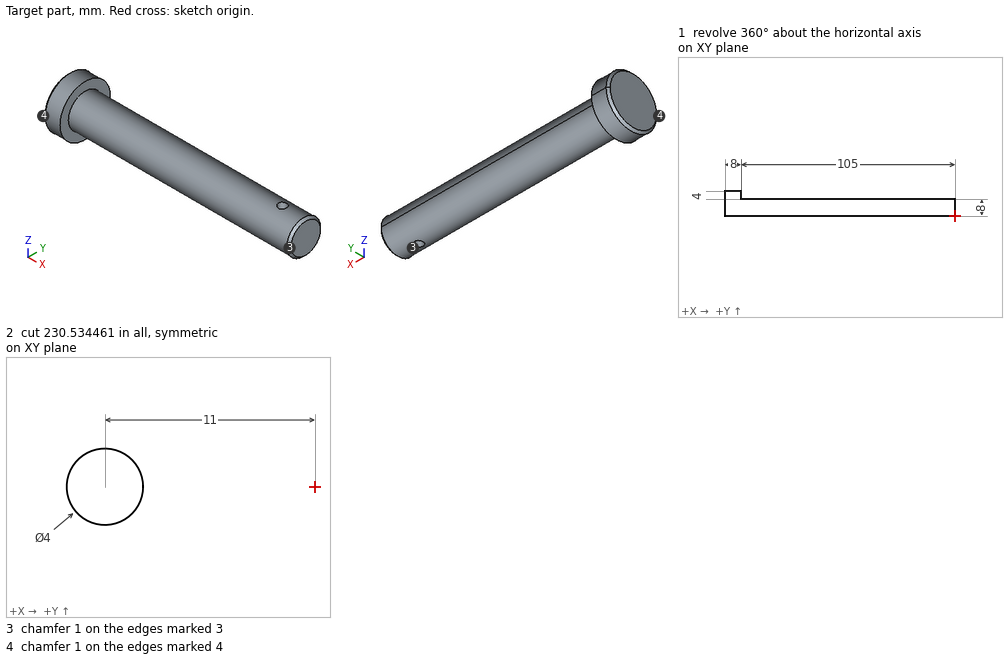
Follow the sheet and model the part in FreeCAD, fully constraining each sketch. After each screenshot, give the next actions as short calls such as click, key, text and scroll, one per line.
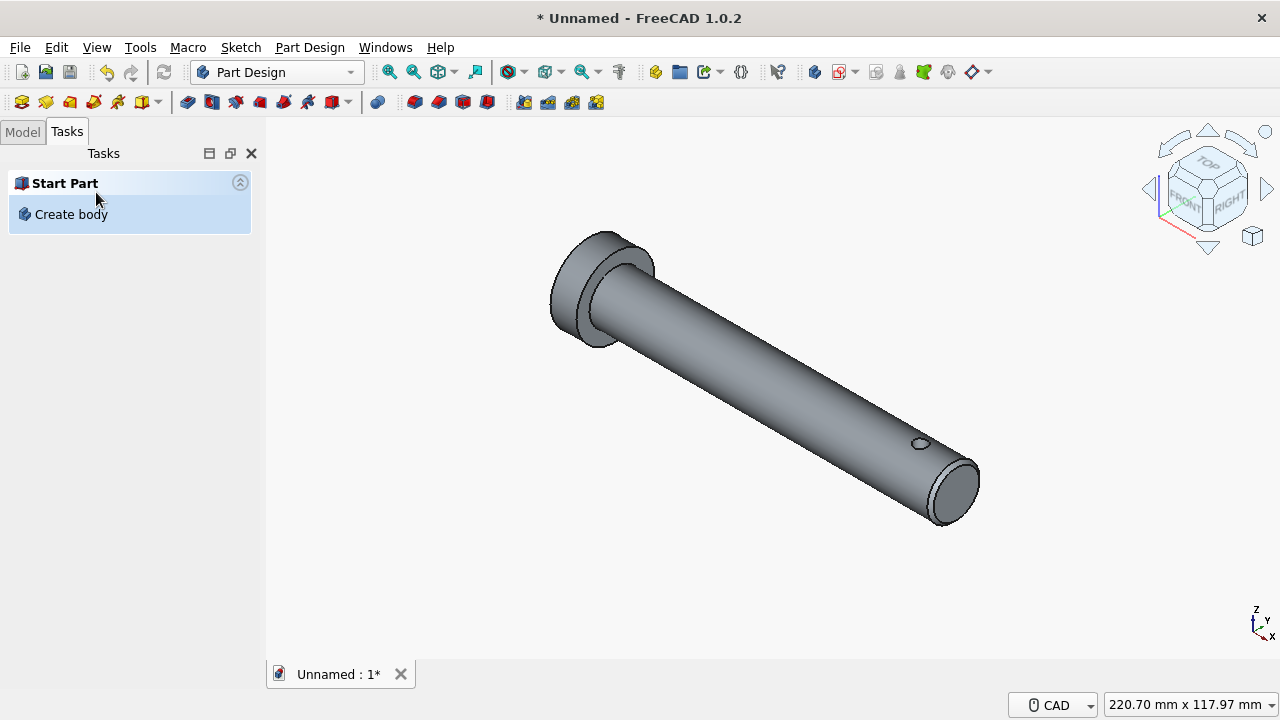
key(2)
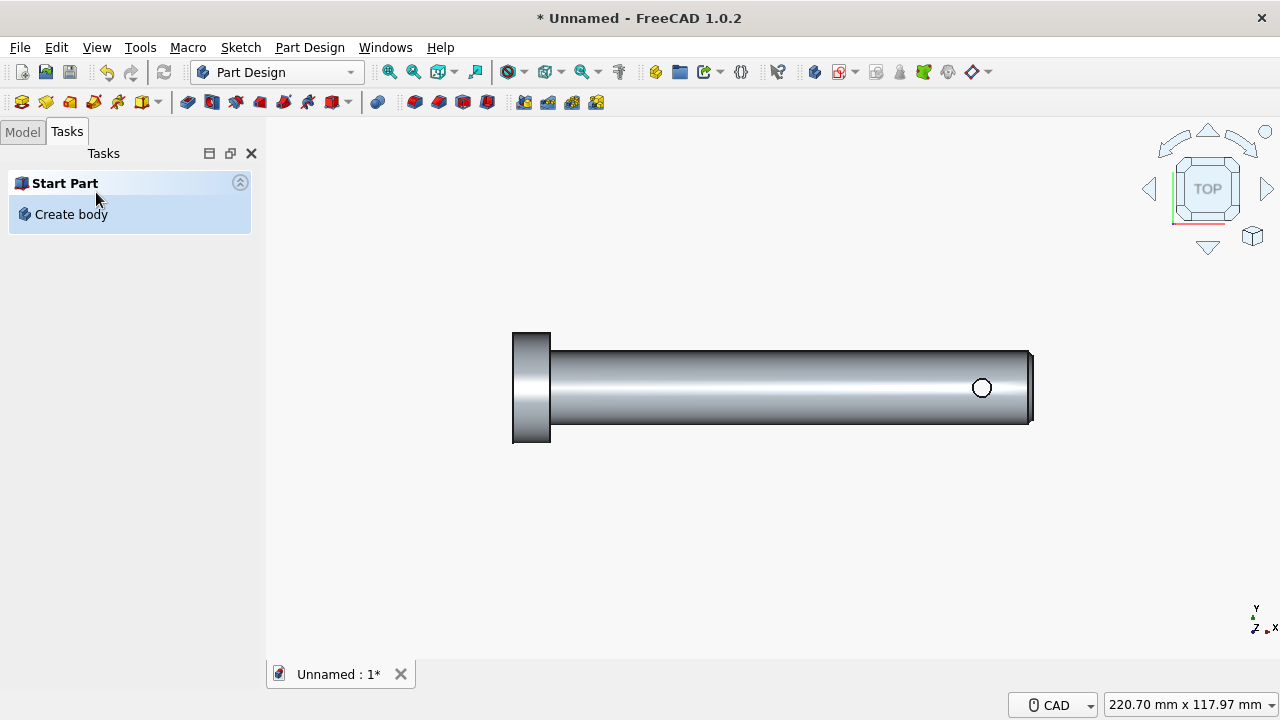
click(513, 432)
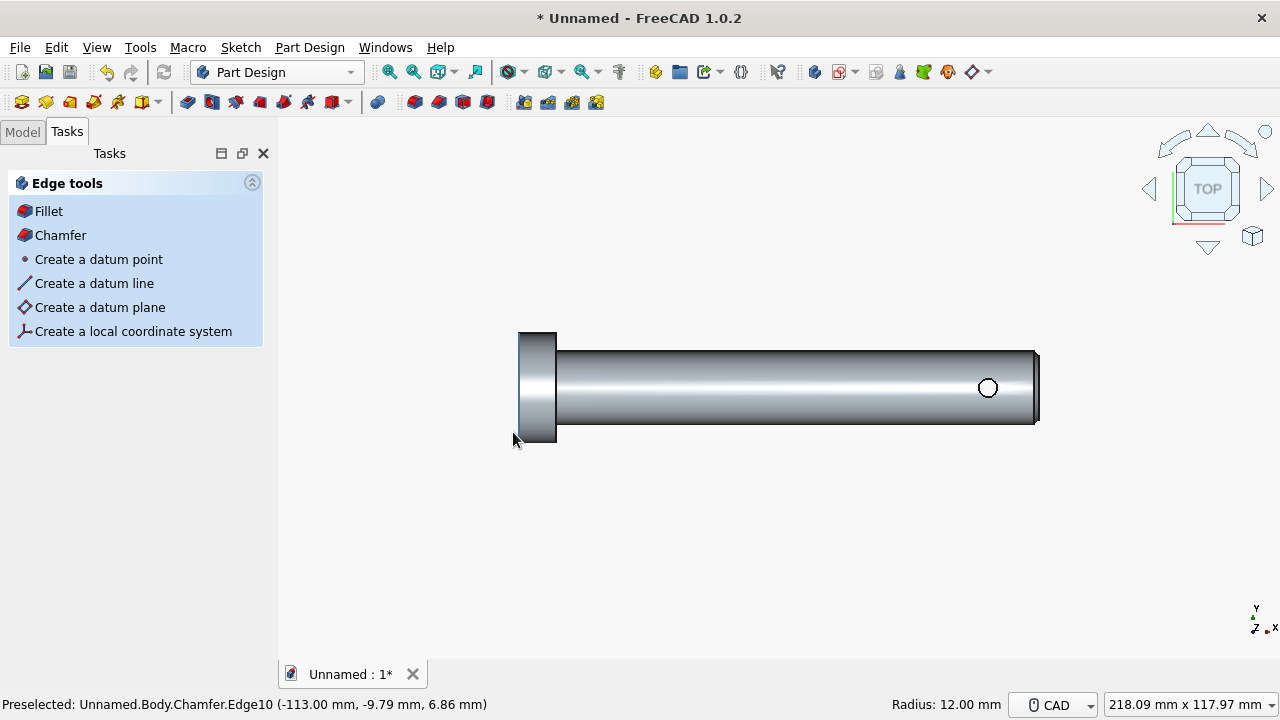
click(440, 102)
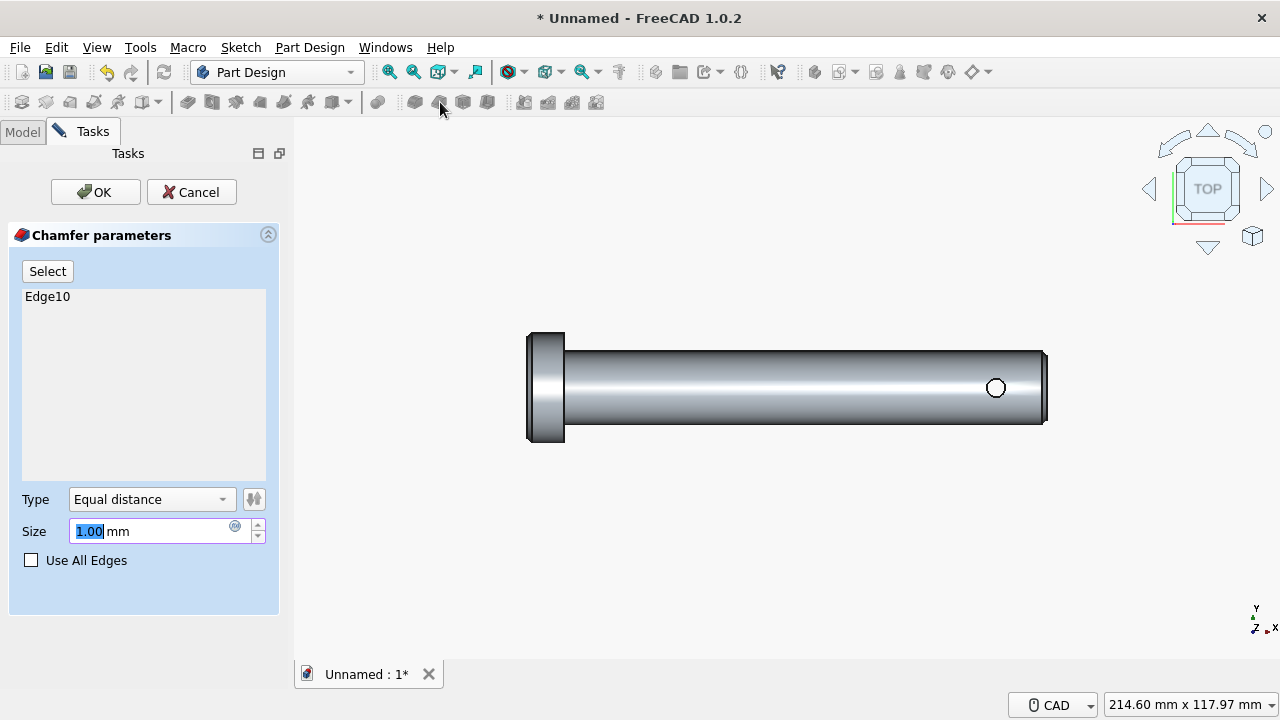
text(1)
key(Tab)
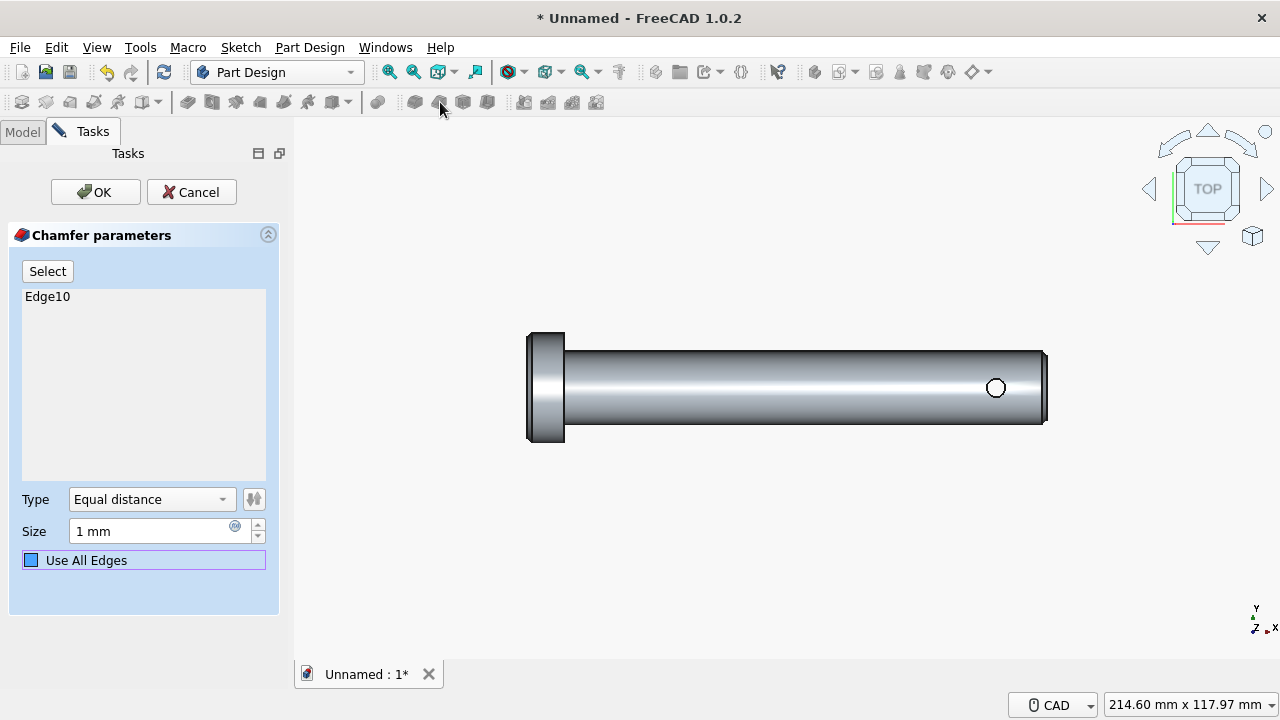
click(96, 192)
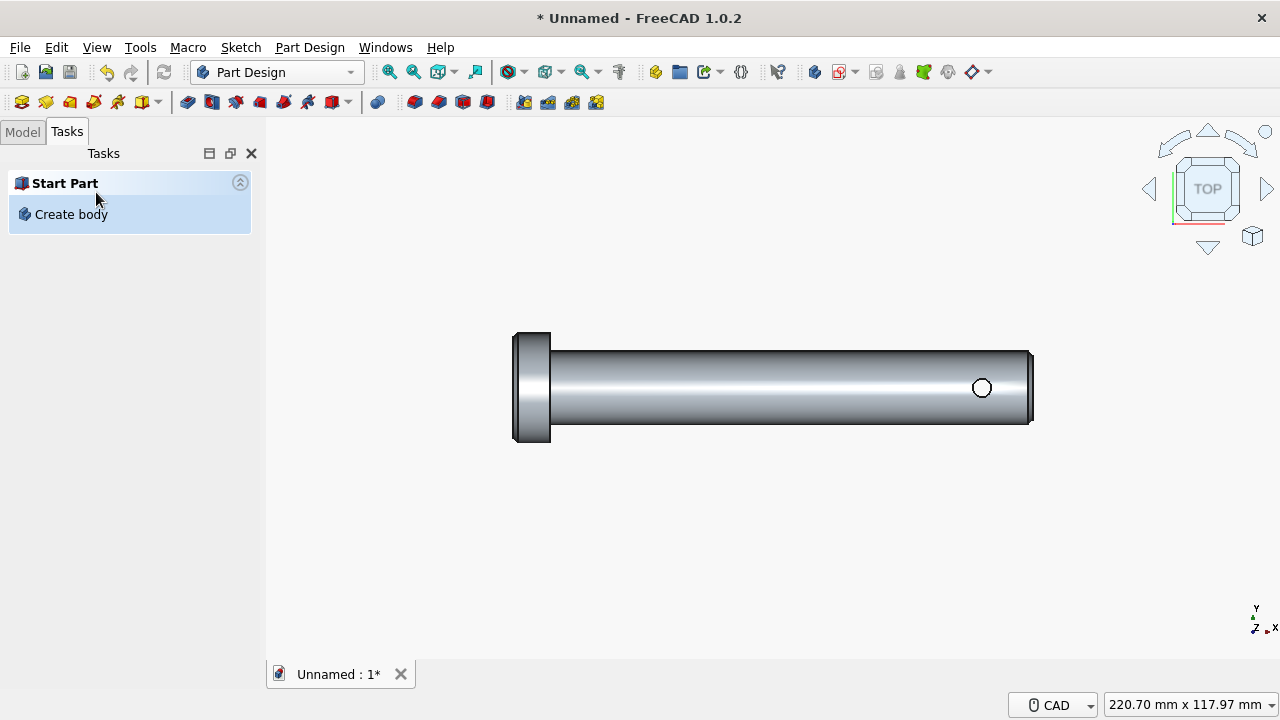
key(0)